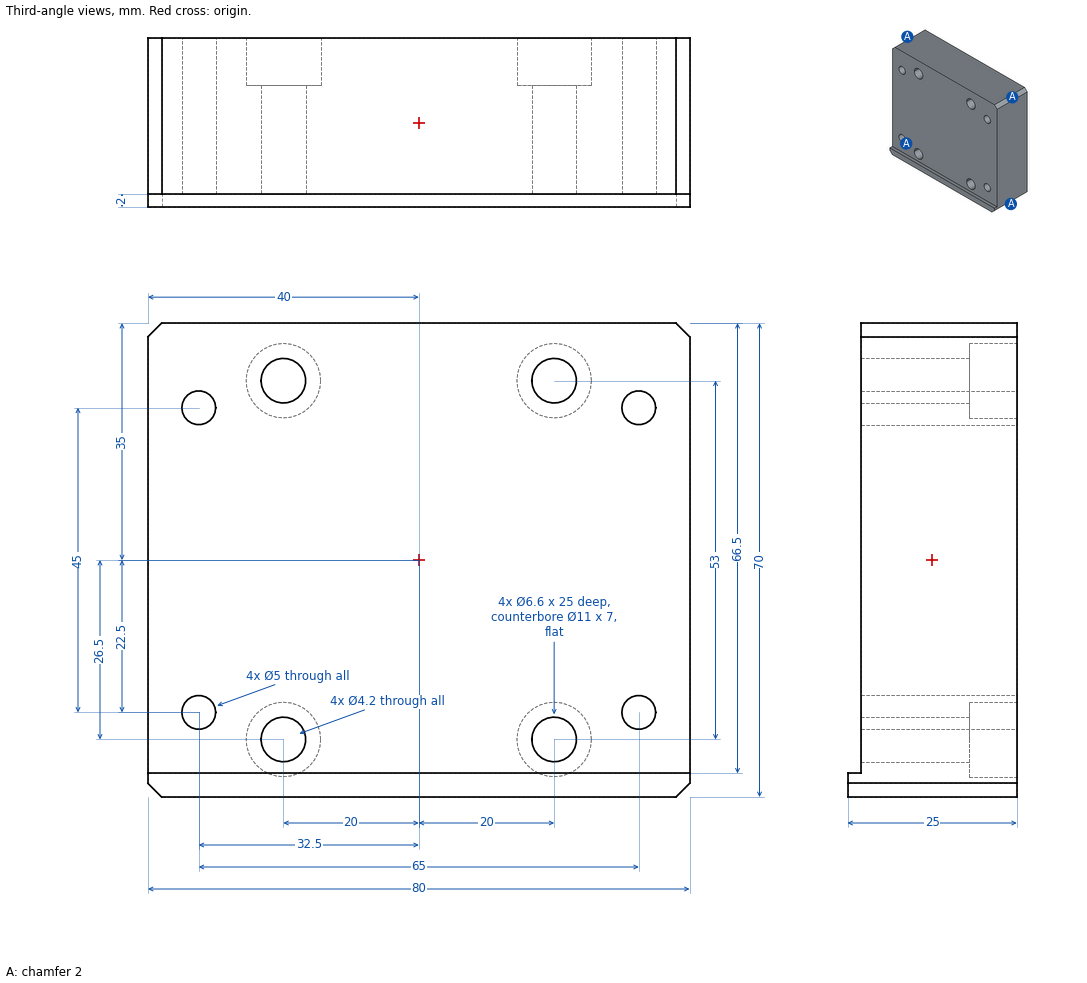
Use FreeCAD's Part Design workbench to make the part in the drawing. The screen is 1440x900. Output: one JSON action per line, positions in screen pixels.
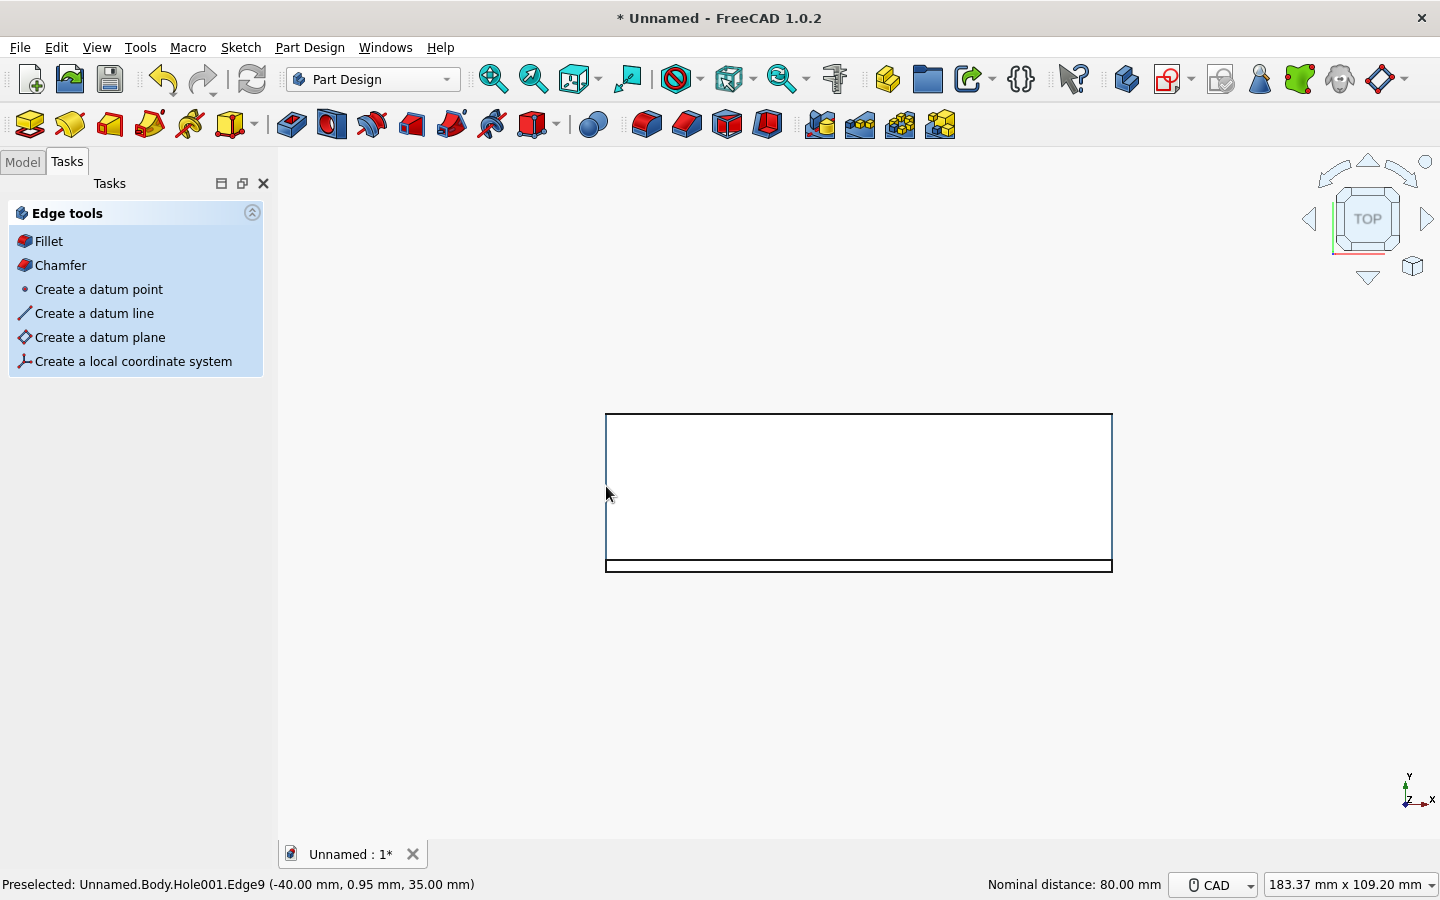
{"action": "key", "text": "1"}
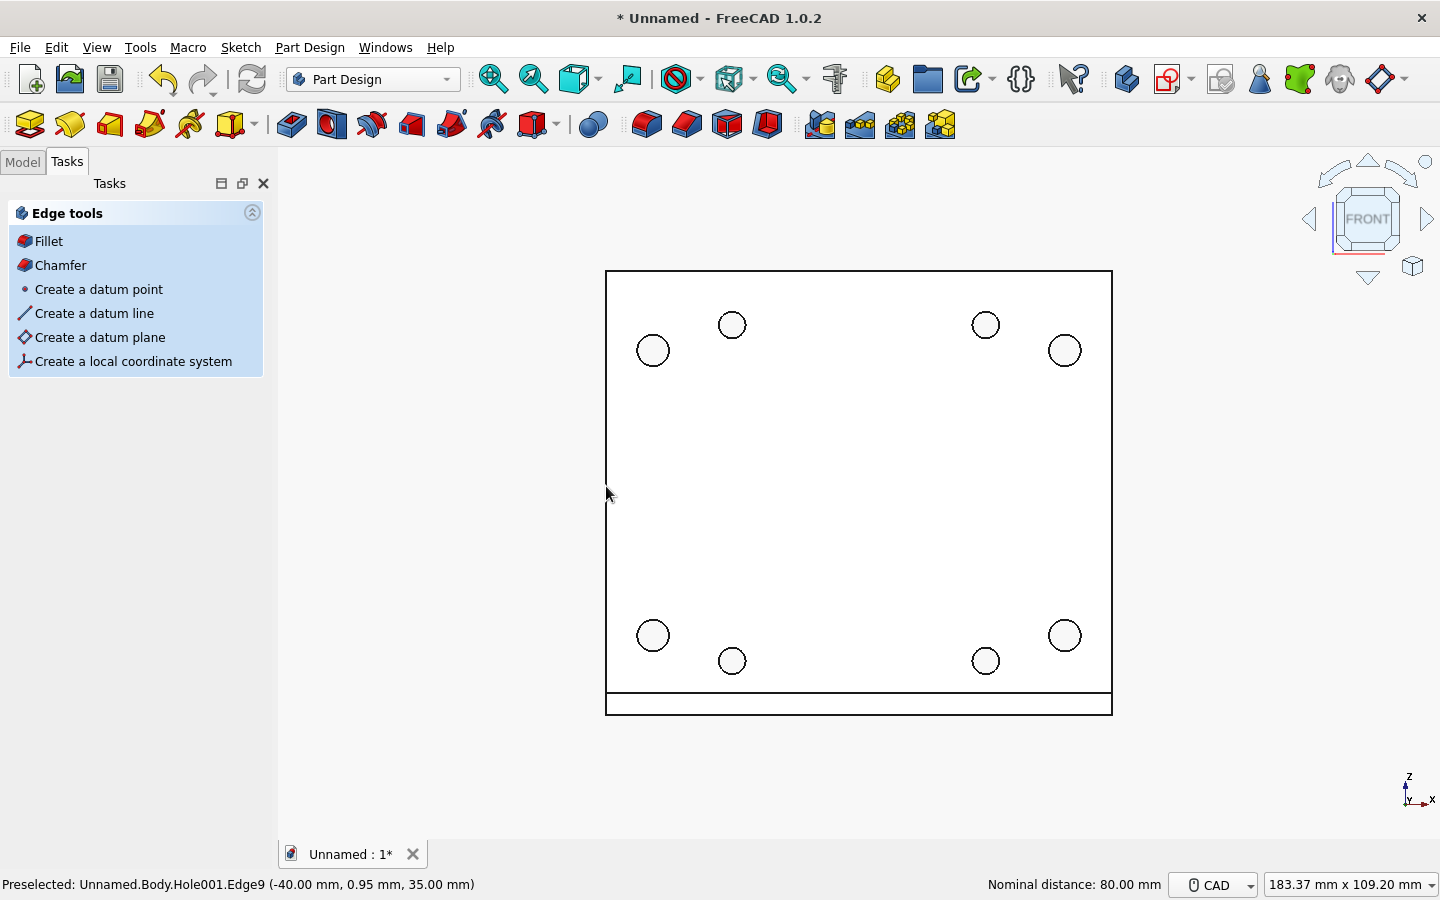
{"action": "key", "text": "3"}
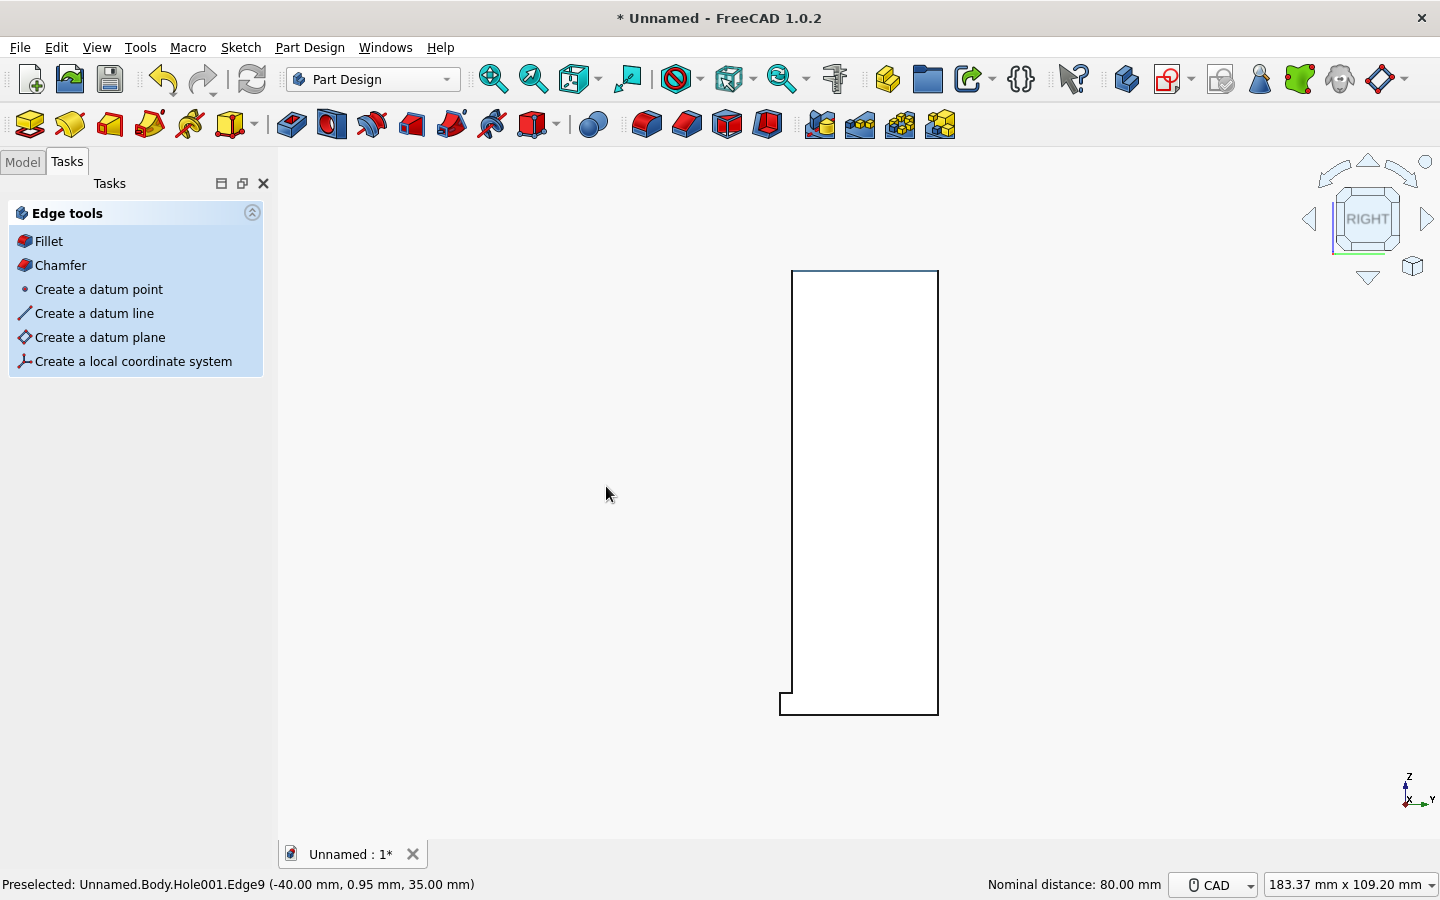
{"action": "left_click", "coordinate": [859, 714], "text": "ctrl"}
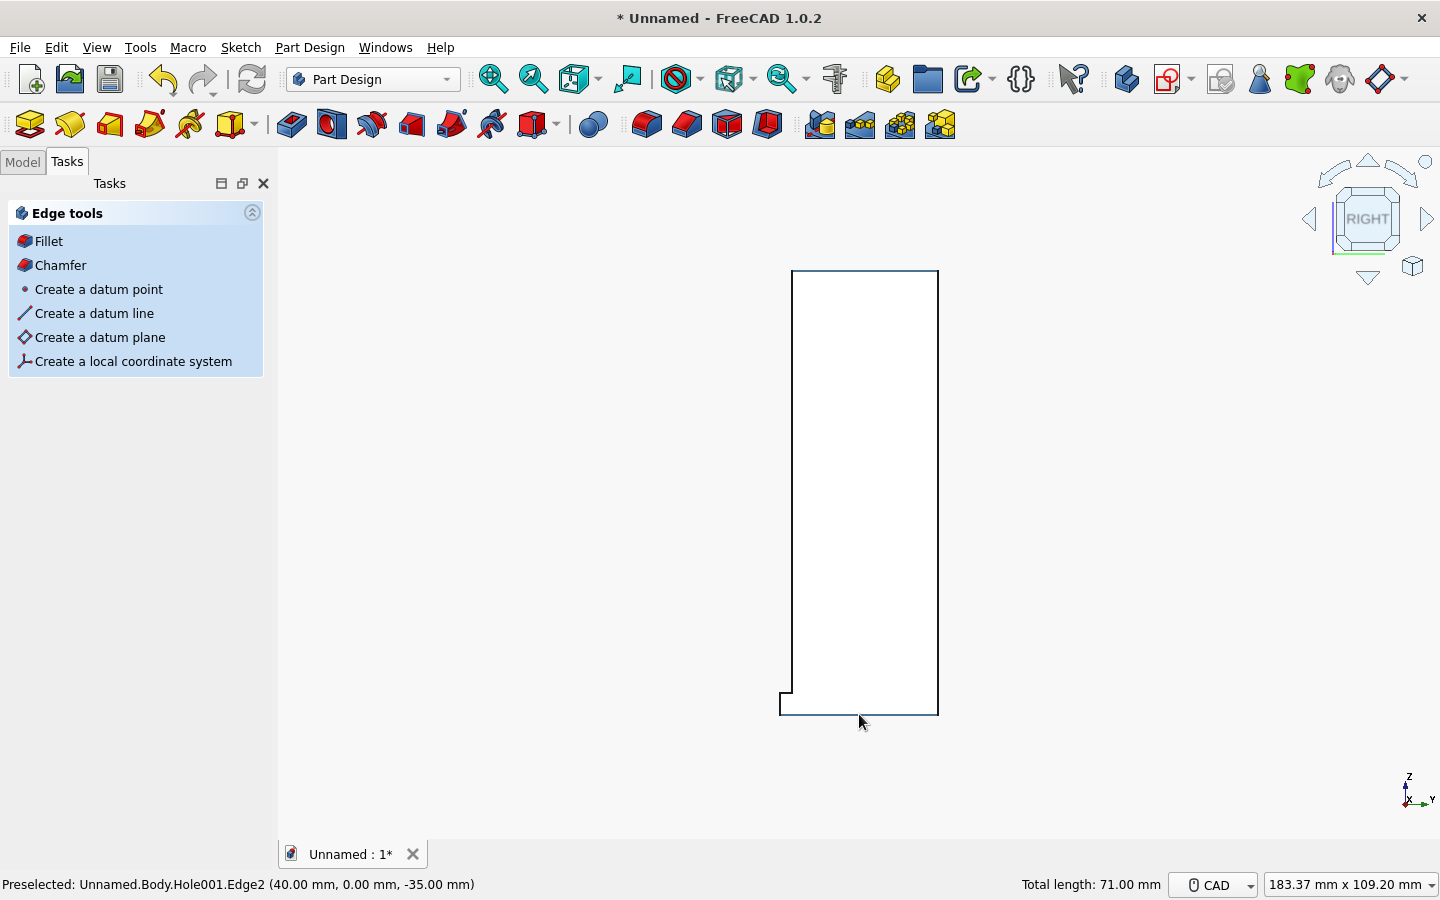
{"action": "key", "text": "5"}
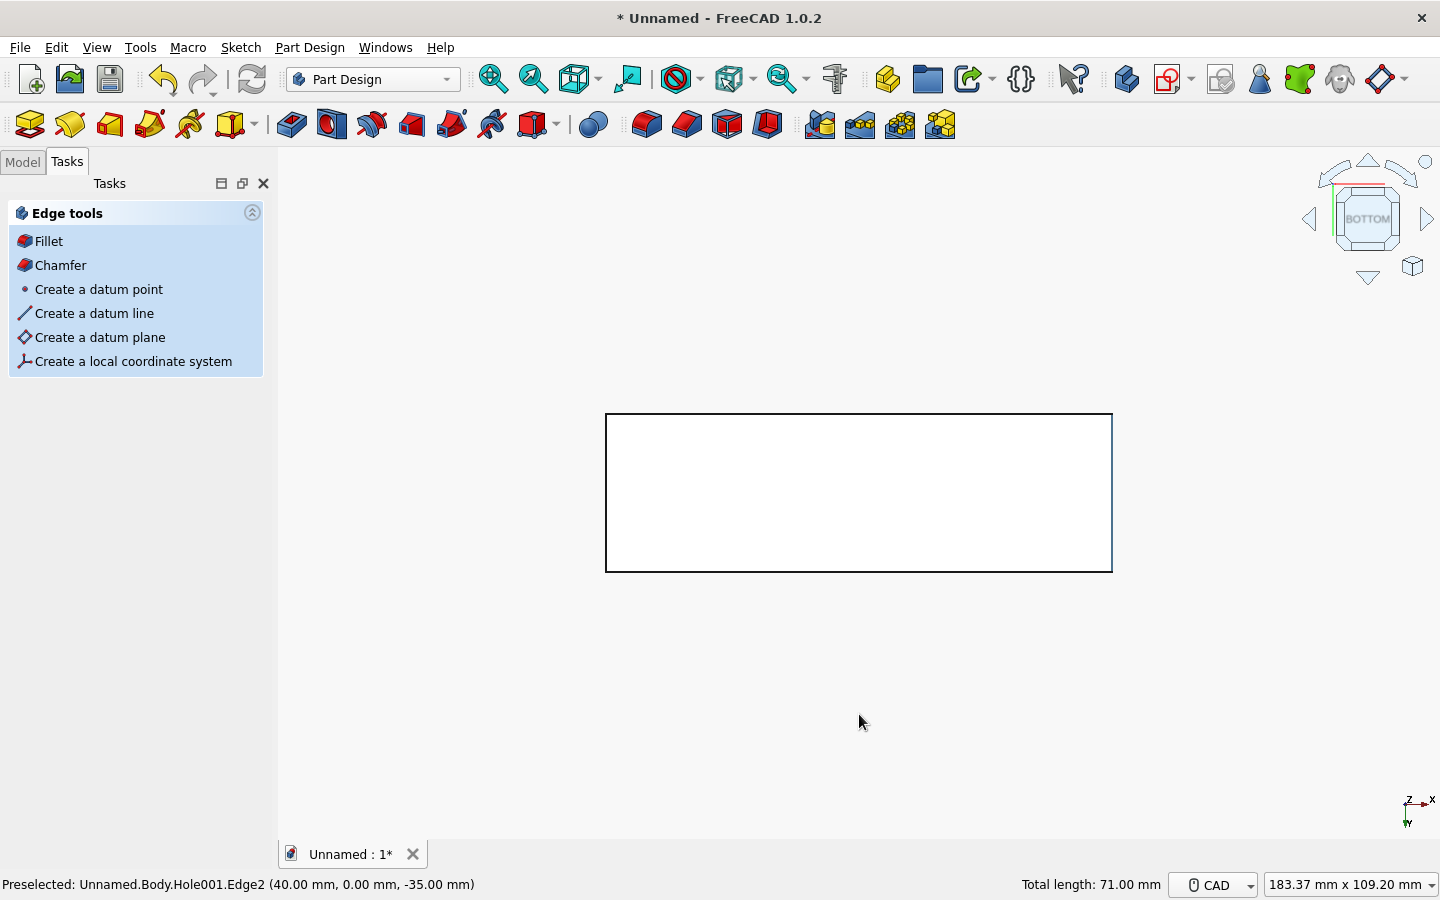
{"action": "left_click", "coordinate": [494, 80]}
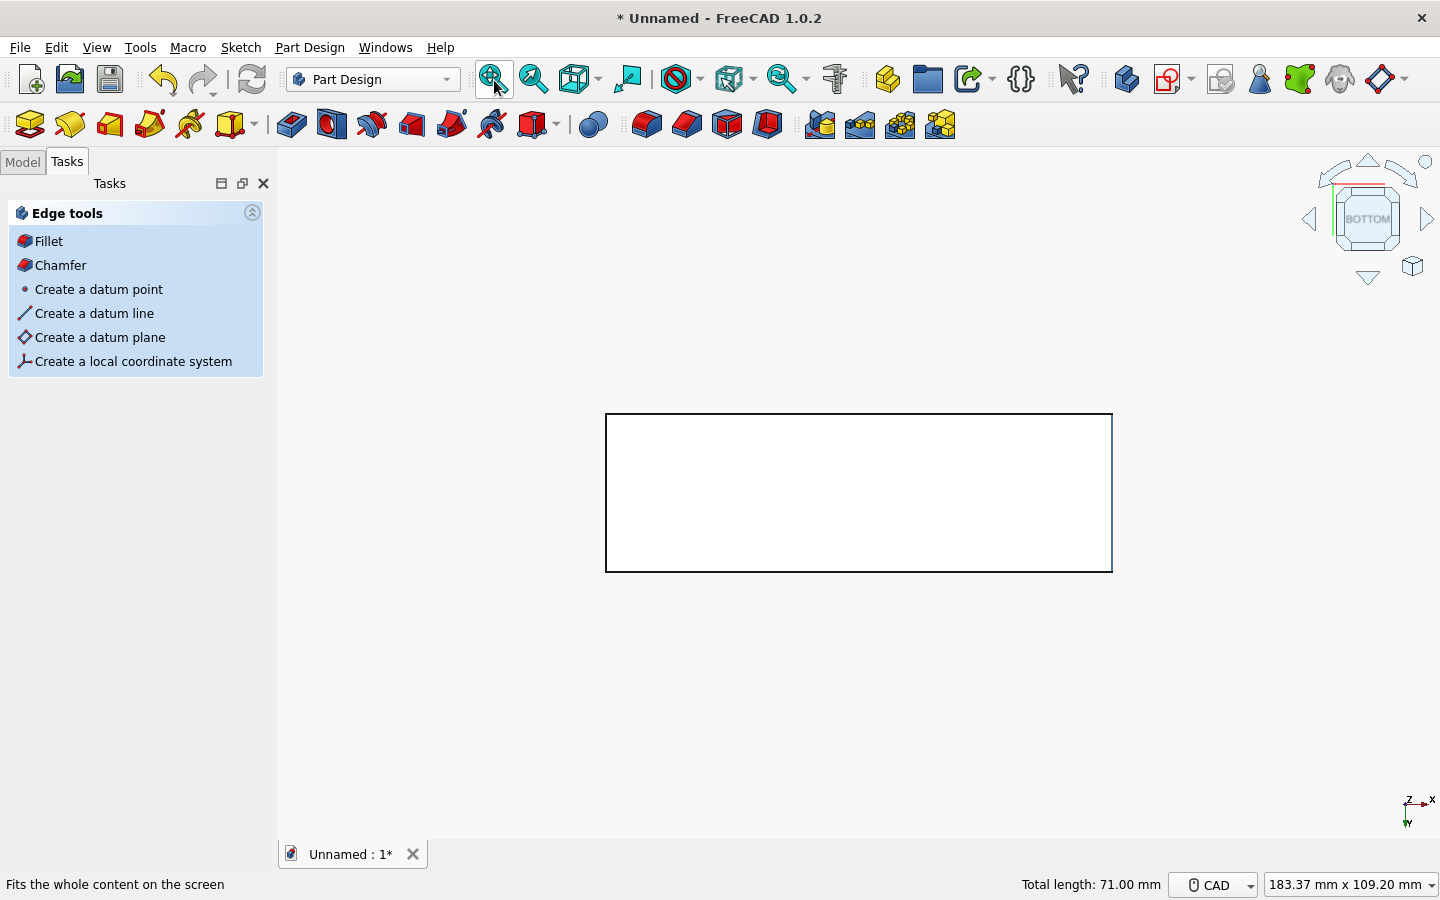
{"action": "left_click", "coordinate": [606, 492], "text": "ctrl"}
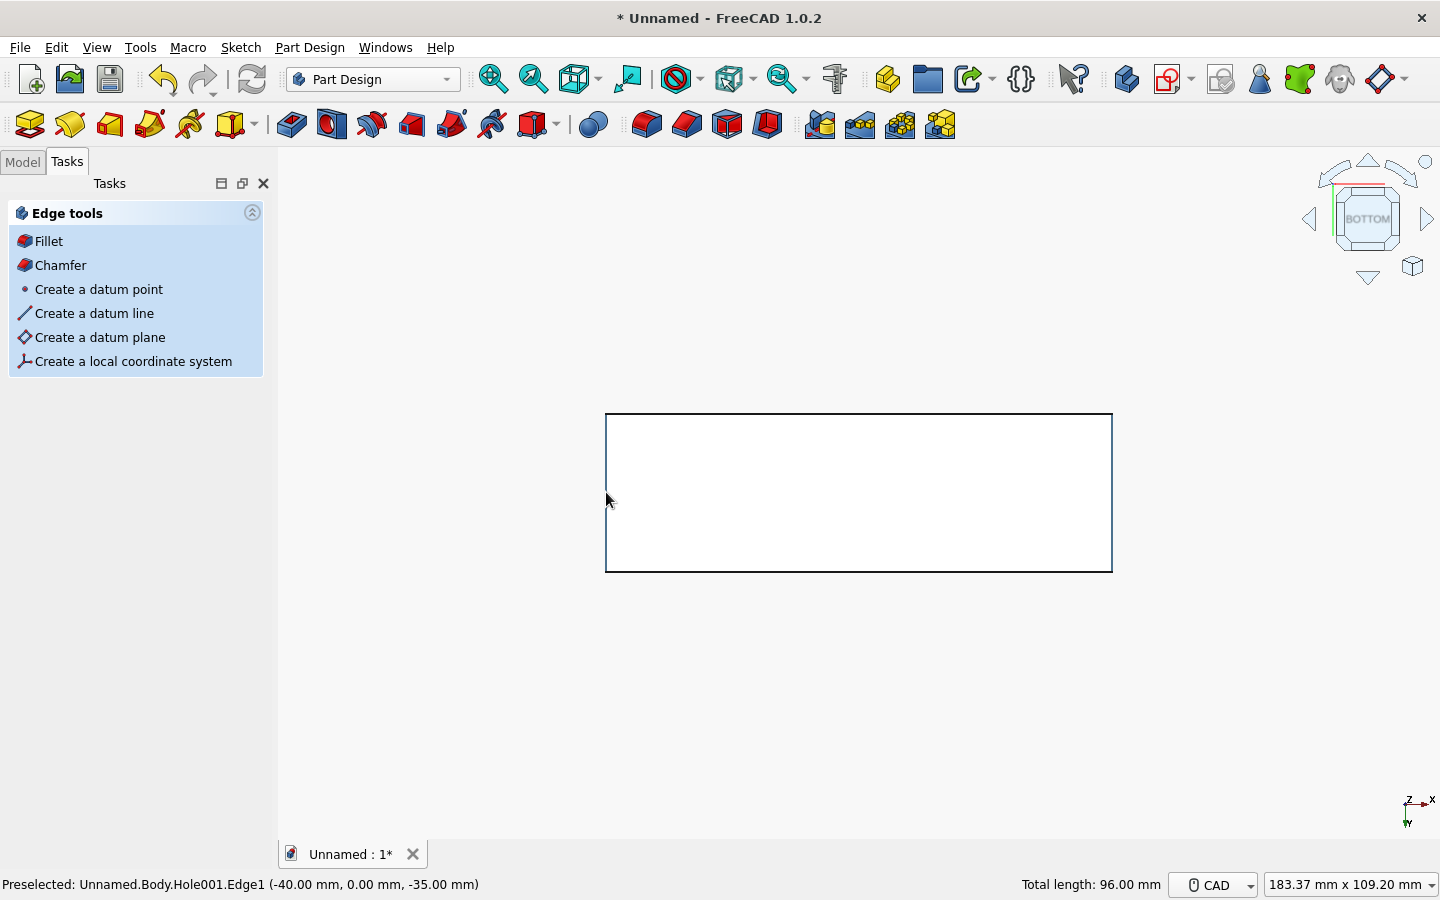
{"action": "left_click", "coordinate": [688, 124]}